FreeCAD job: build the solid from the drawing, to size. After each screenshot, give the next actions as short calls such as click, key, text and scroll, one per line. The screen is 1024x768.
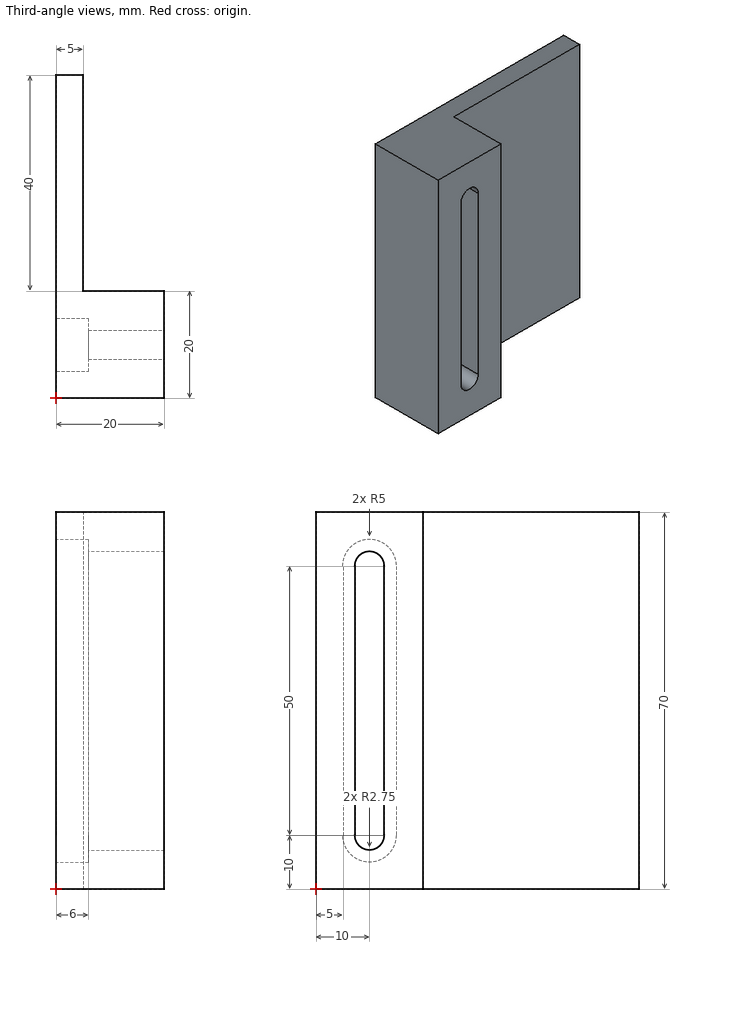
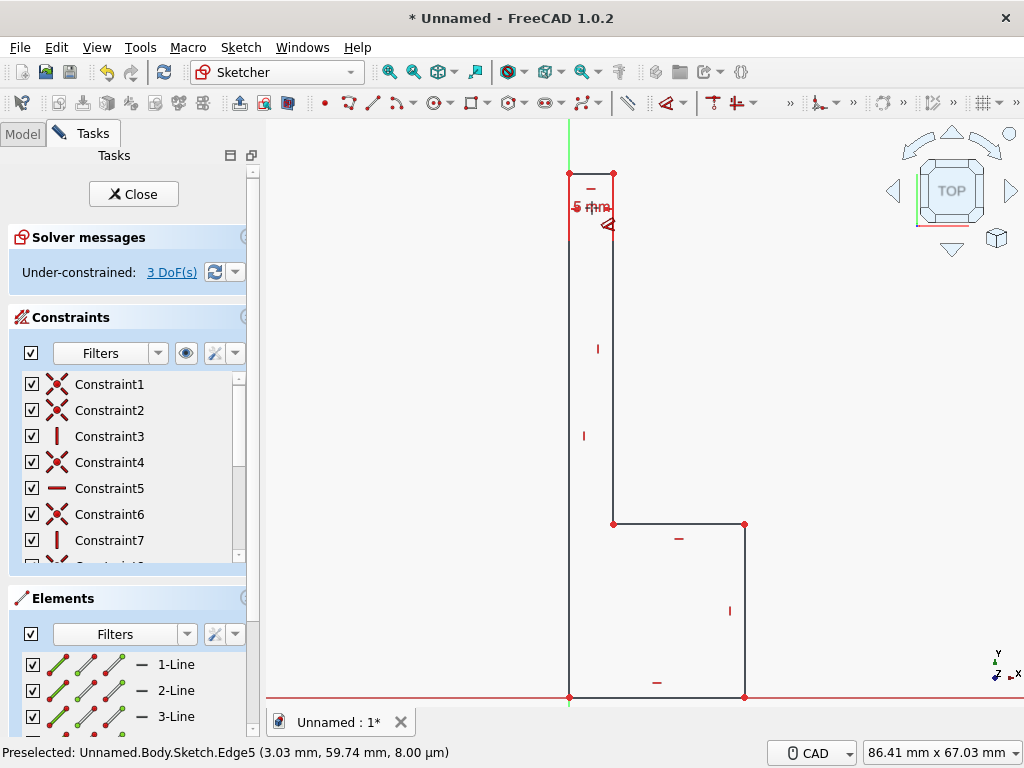
scroll(413, 369, down, 2)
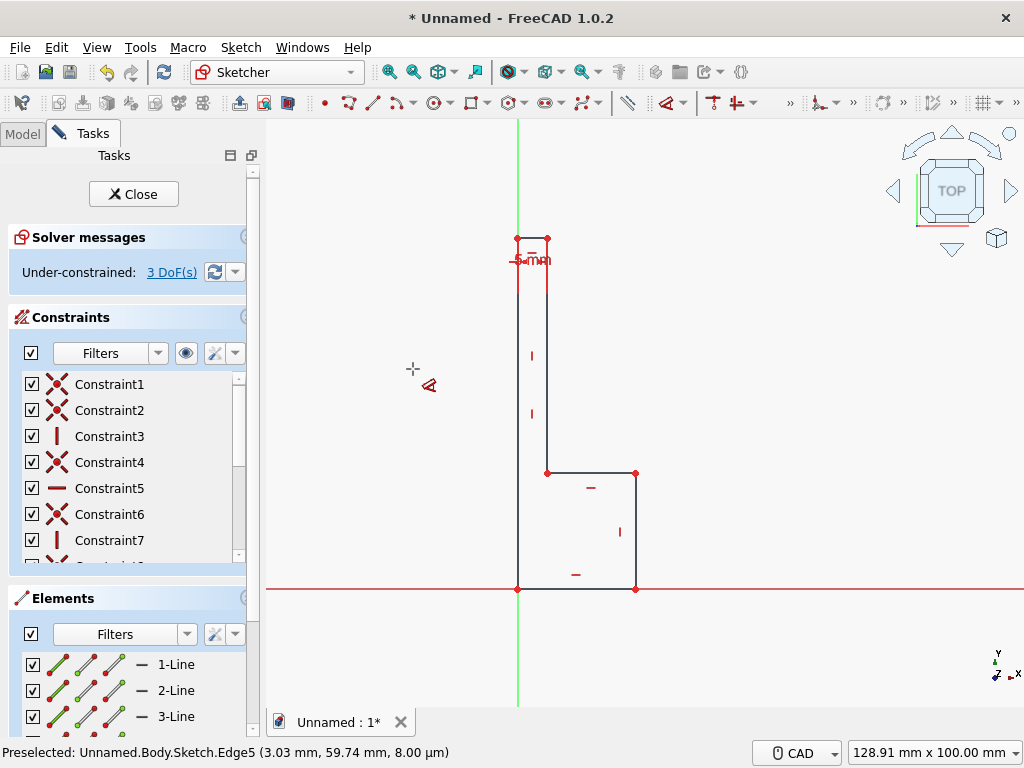
click(553, 589)
click(577, 623)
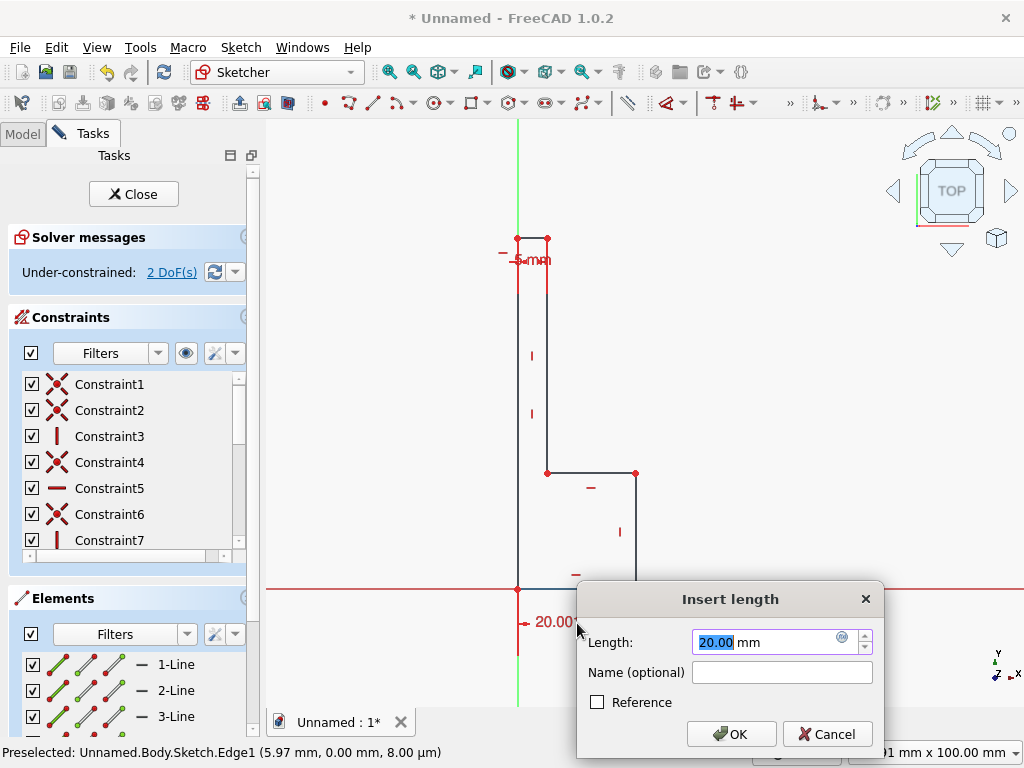
text(20)
key(Return)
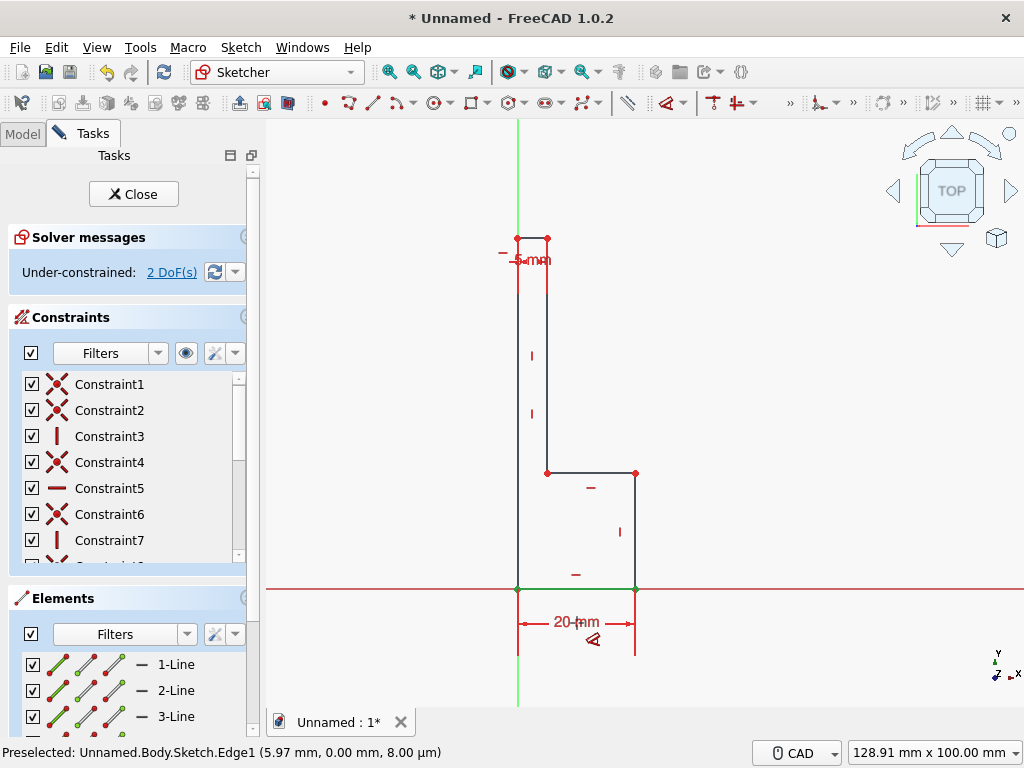
click(636, 555)
click(670, 531)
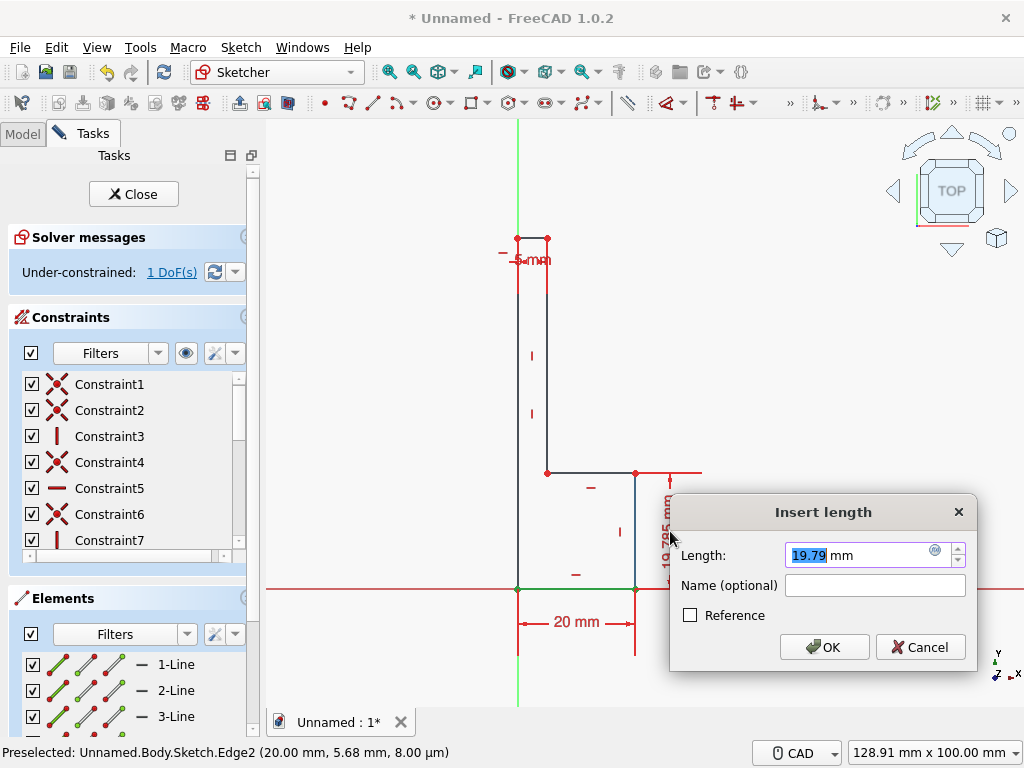
text(20)
key(Return)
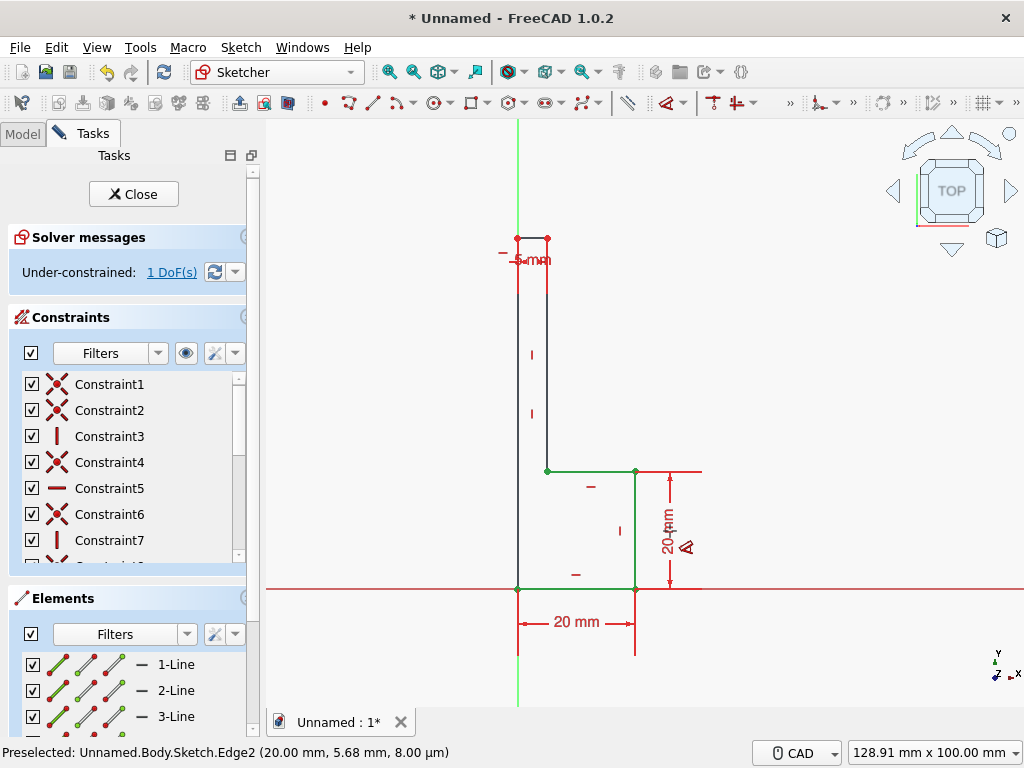
click(547, 402)
click(581, 355)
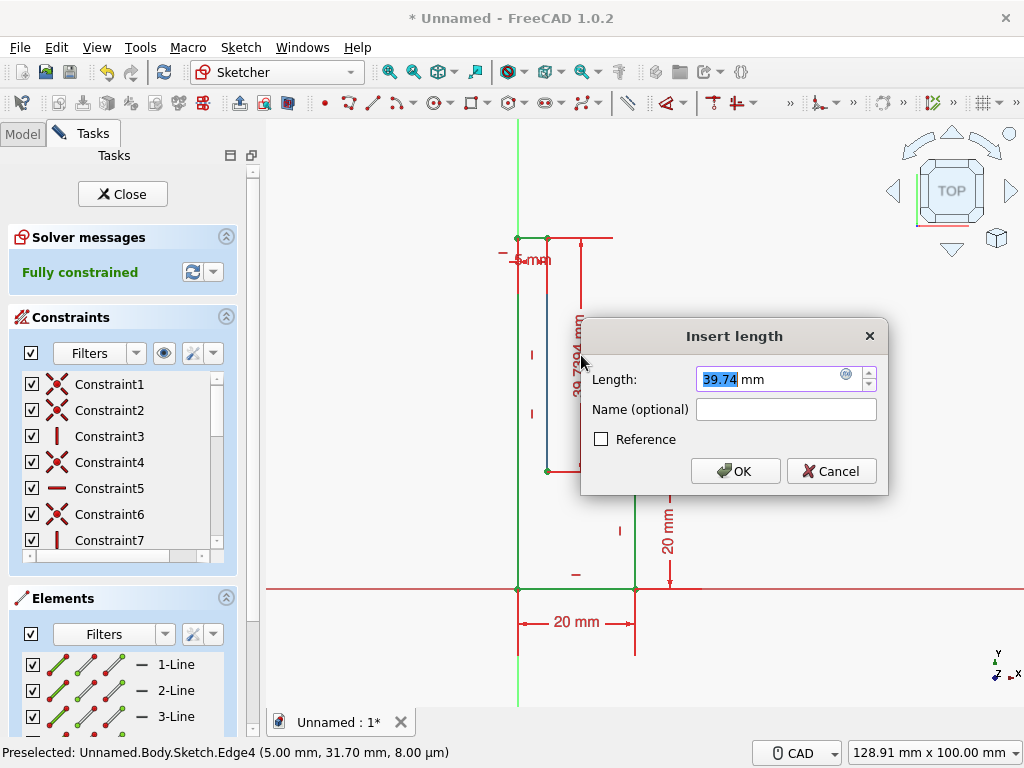
text(40)
key(Return)
key(Escape)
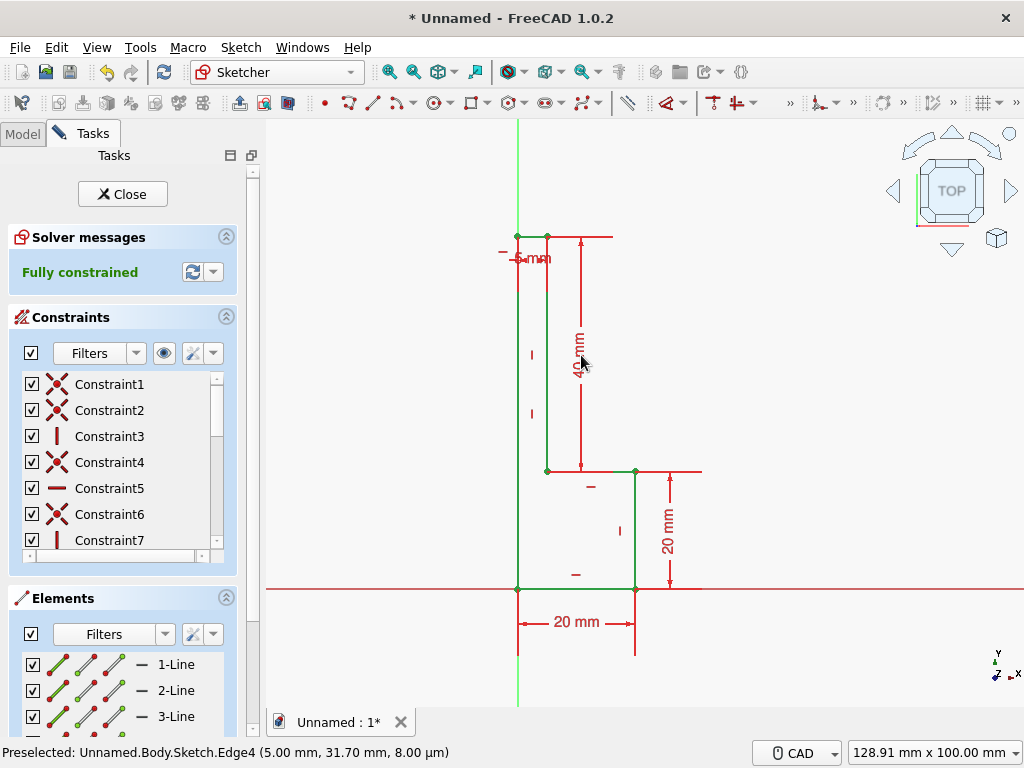
click(123, 194)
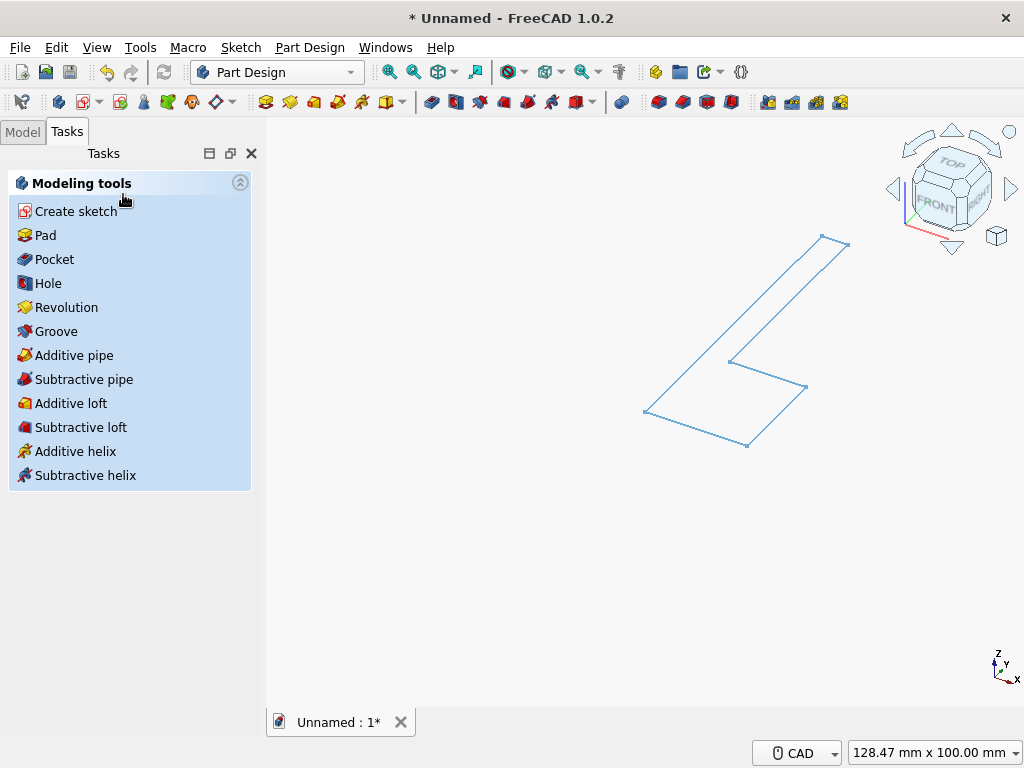
click(266, 102)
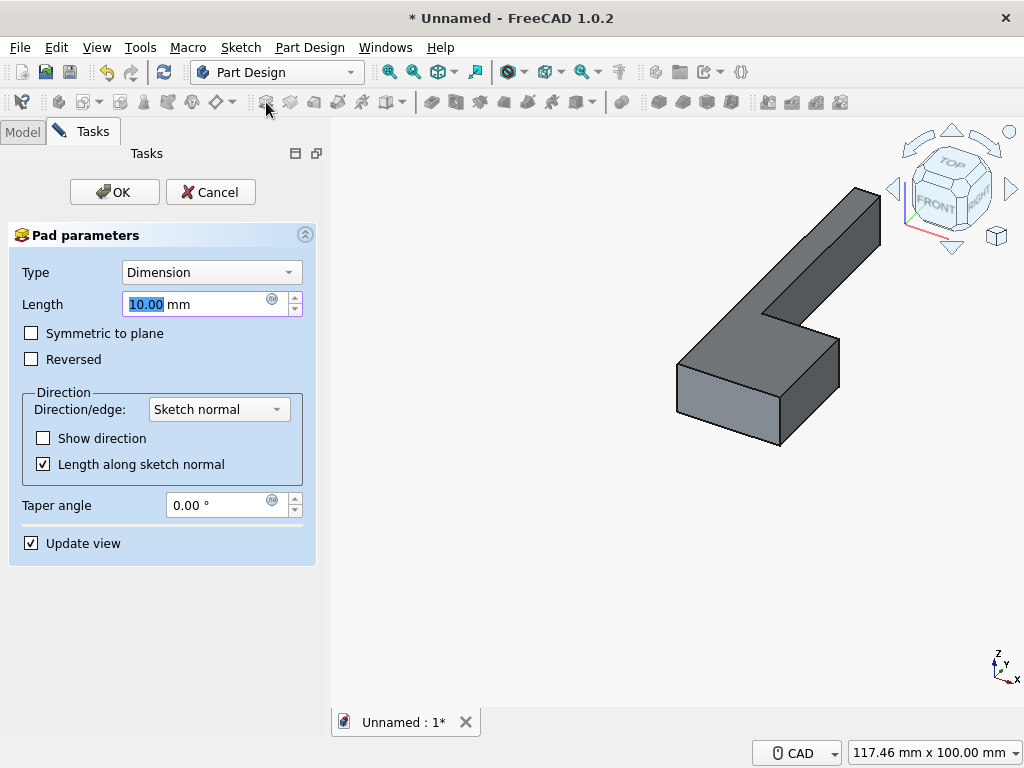
text(70)
key(Tab)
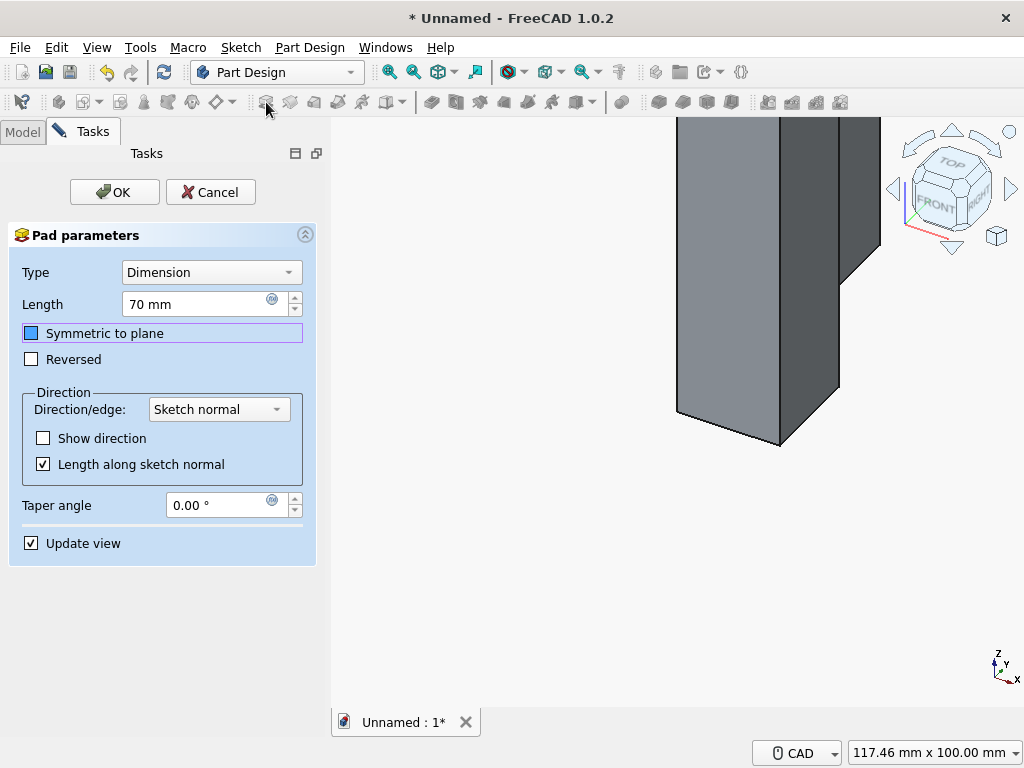
click(115, 192)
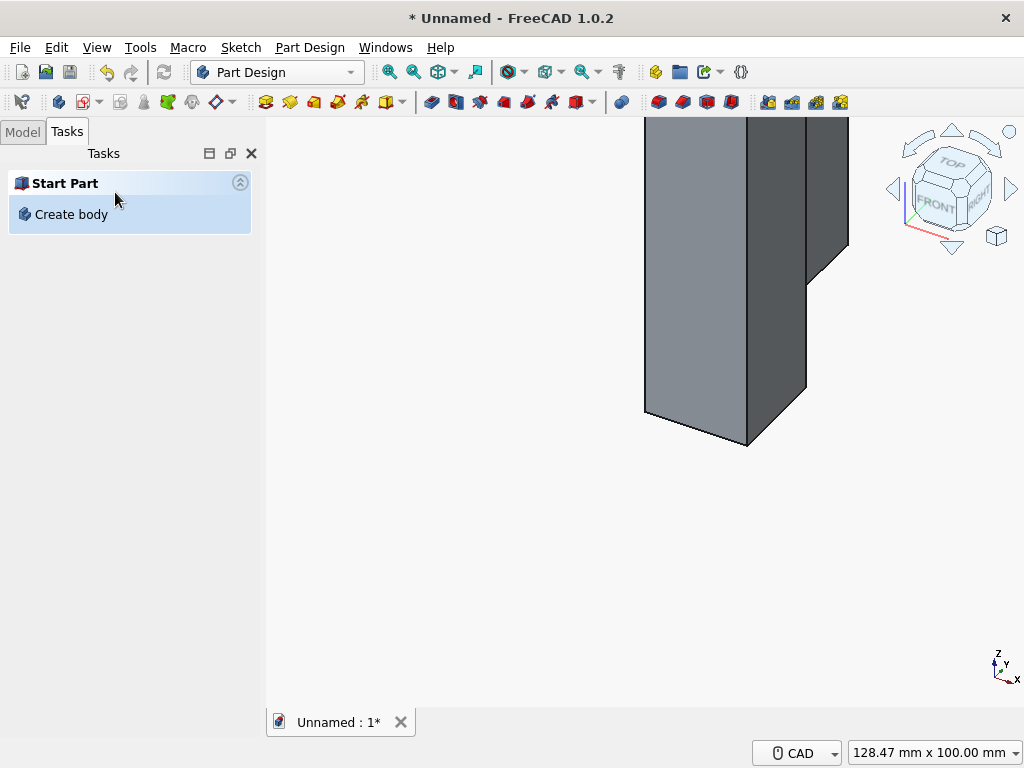
click(390, 72)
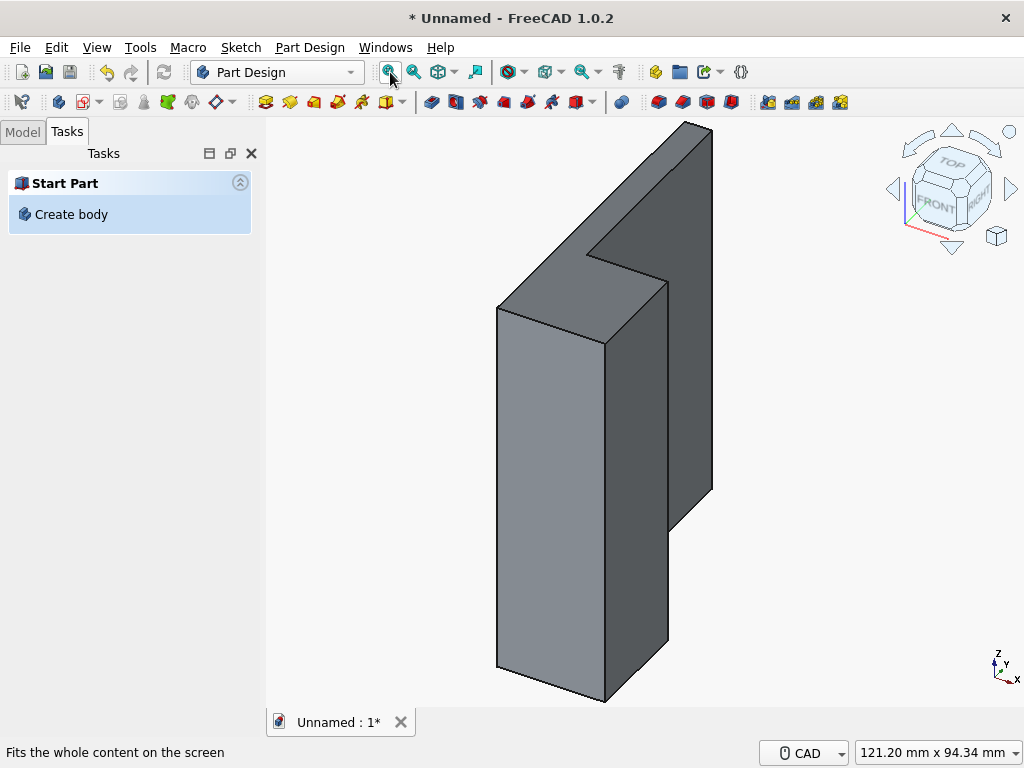
key(6)